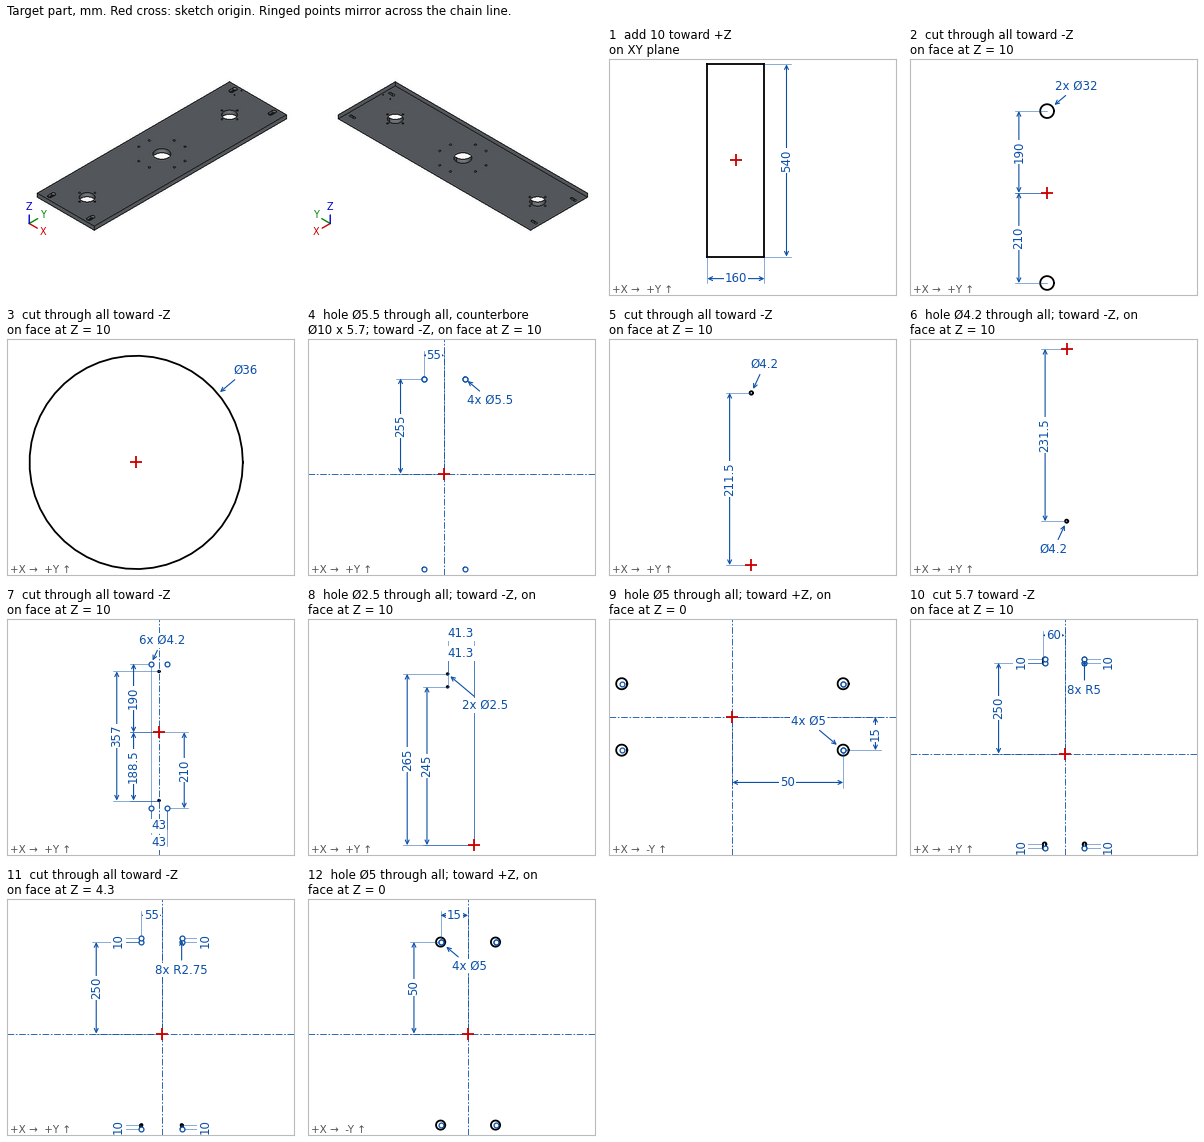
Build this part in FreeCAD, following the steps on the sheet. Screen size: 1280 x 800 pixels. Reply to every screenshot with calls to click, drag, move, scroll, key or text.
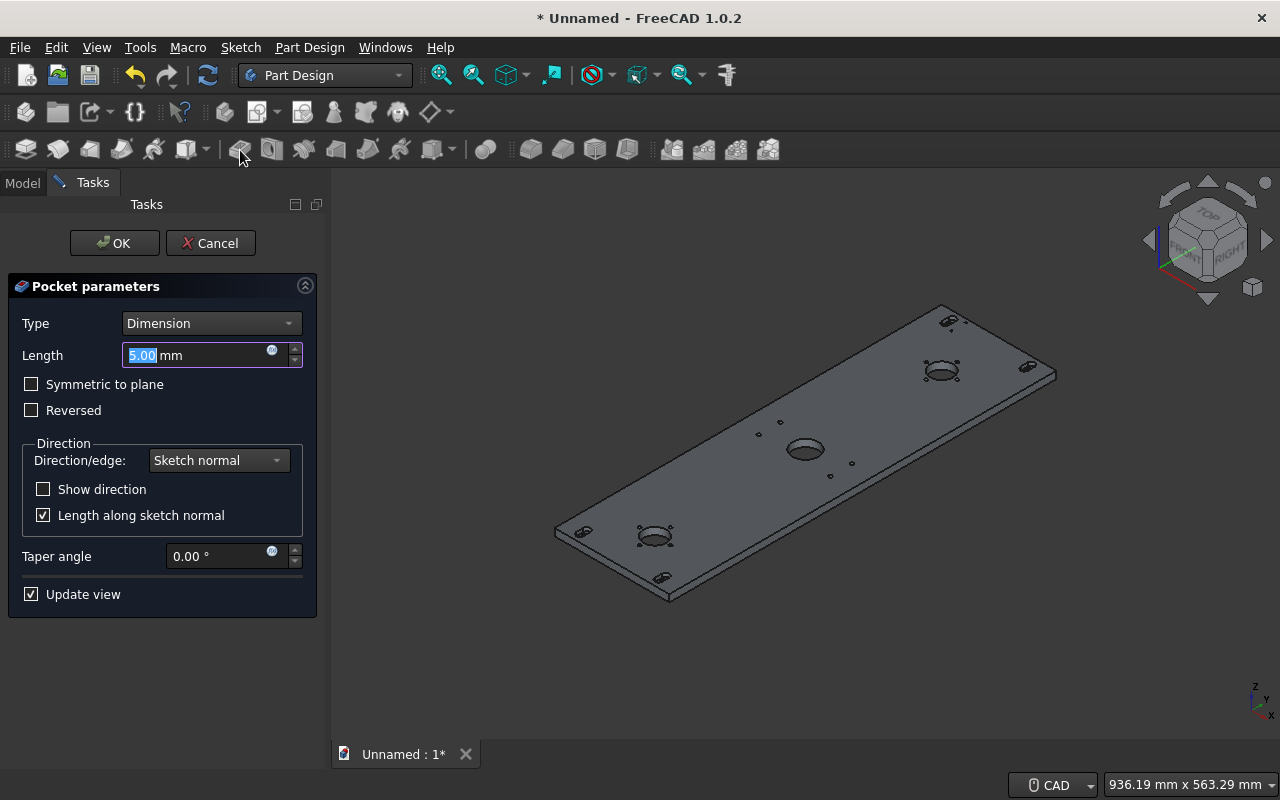
text(5.7)
key(Tab)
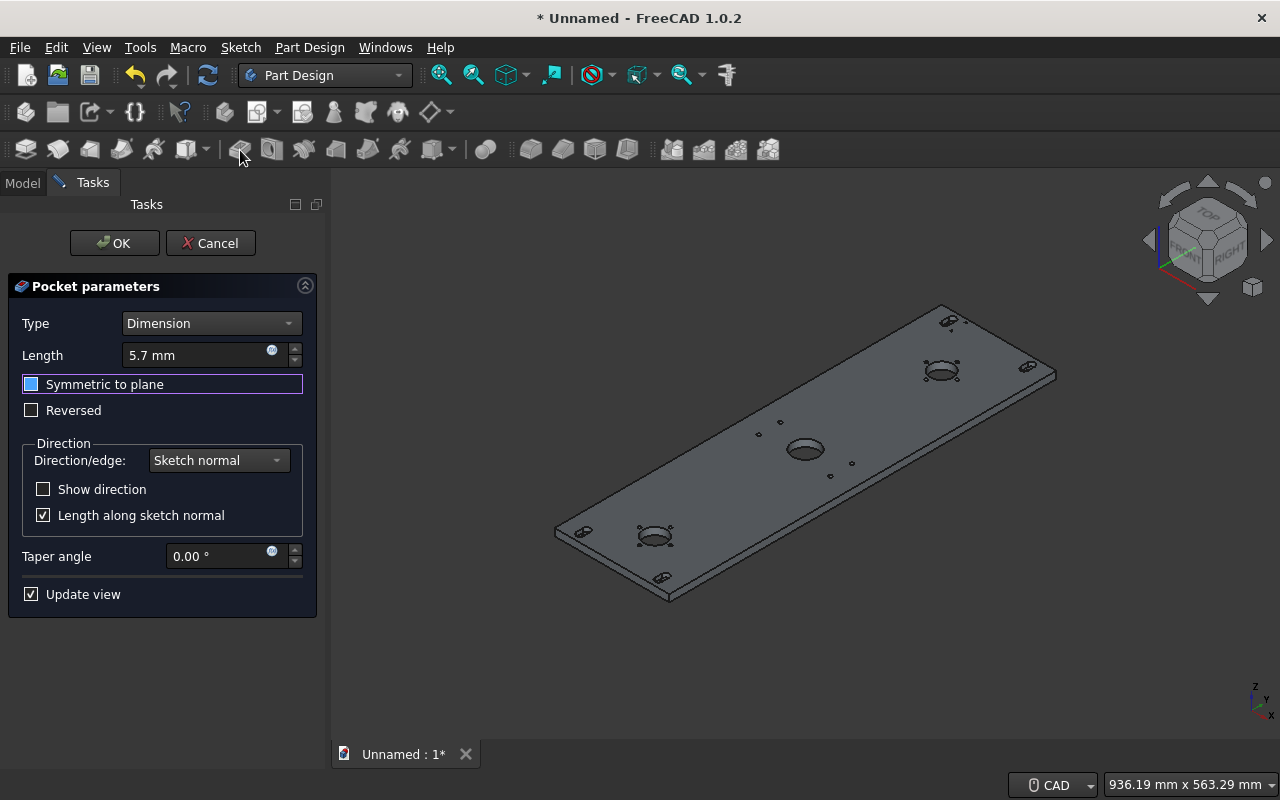
click(115, 243)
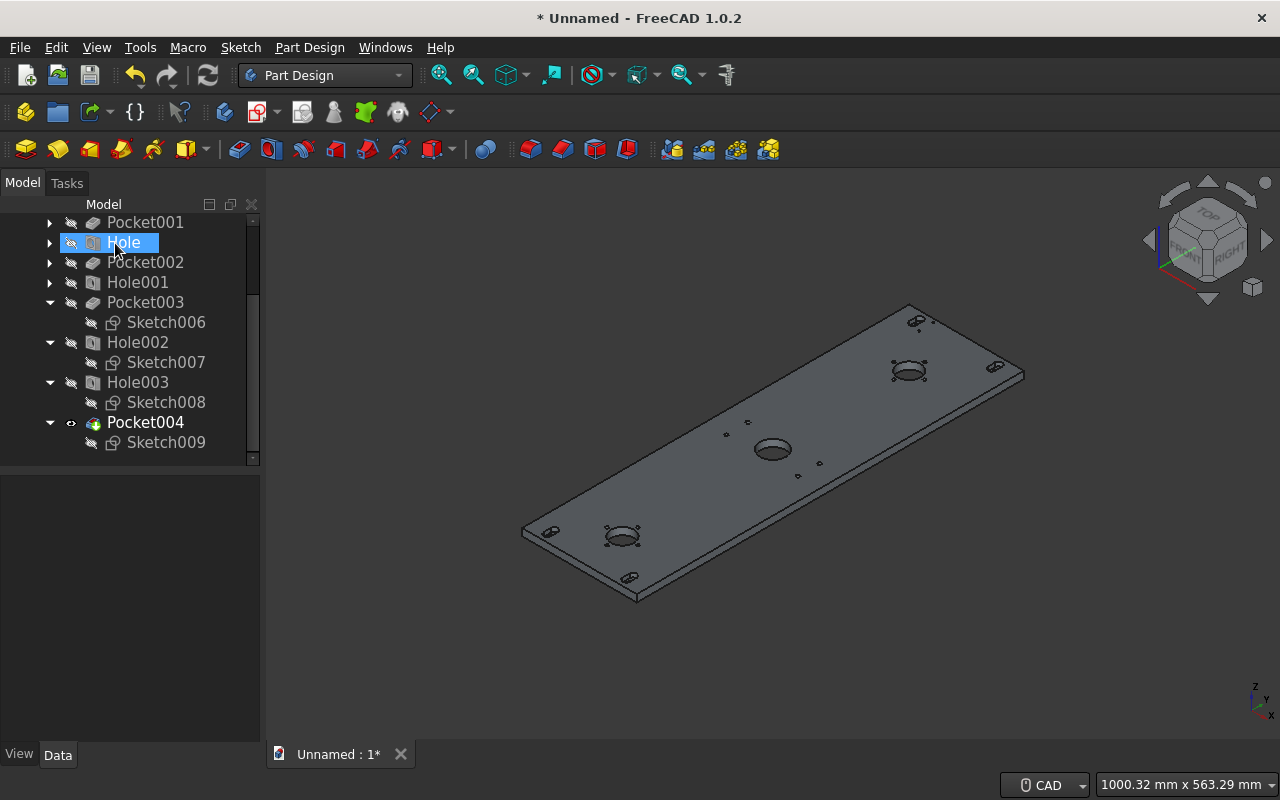
scroll(913, 328, up, 7)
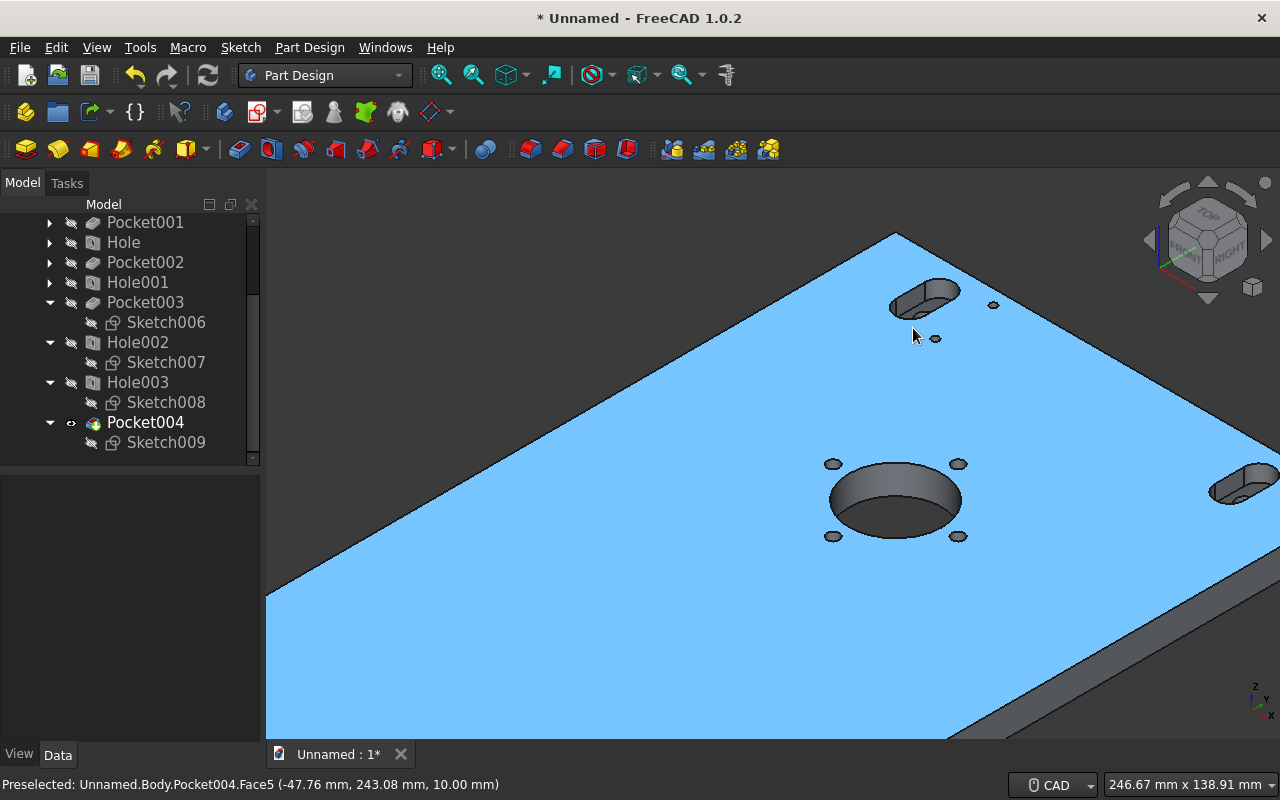
click(442, 76)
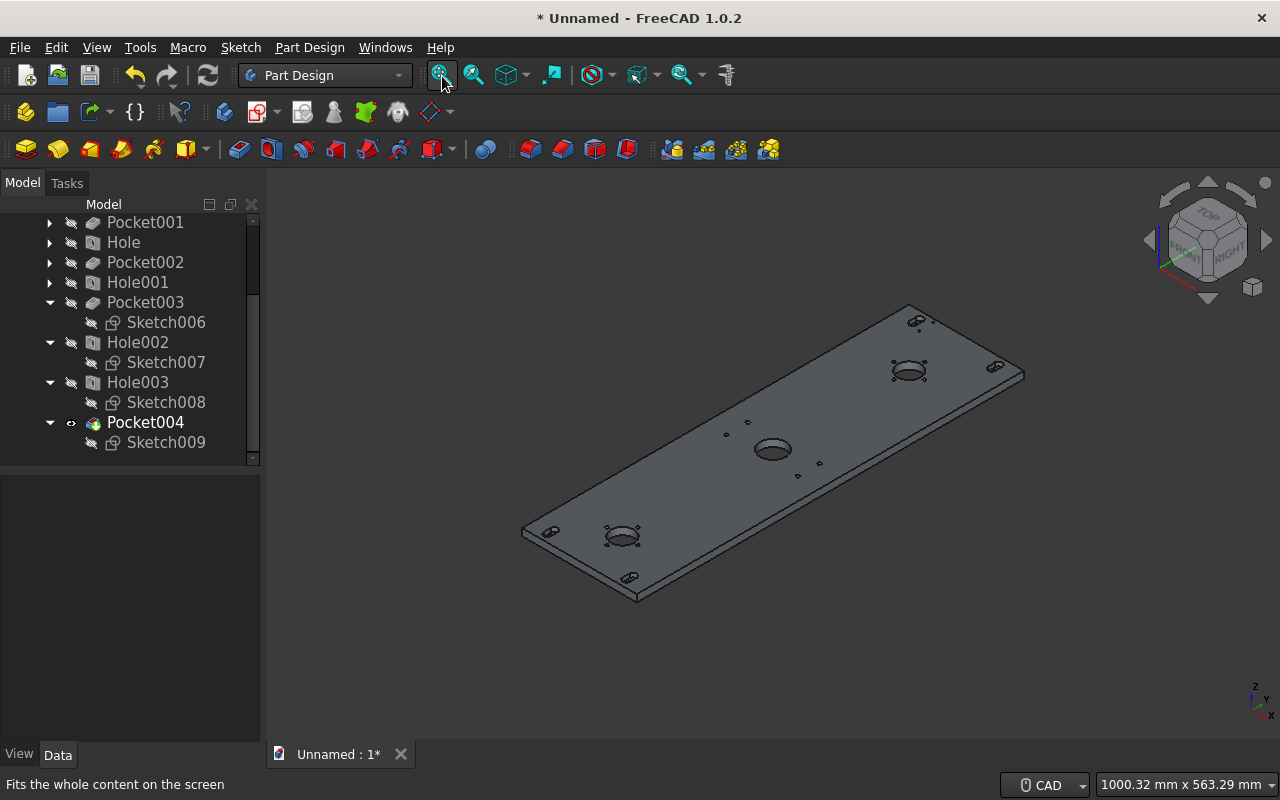
key(2)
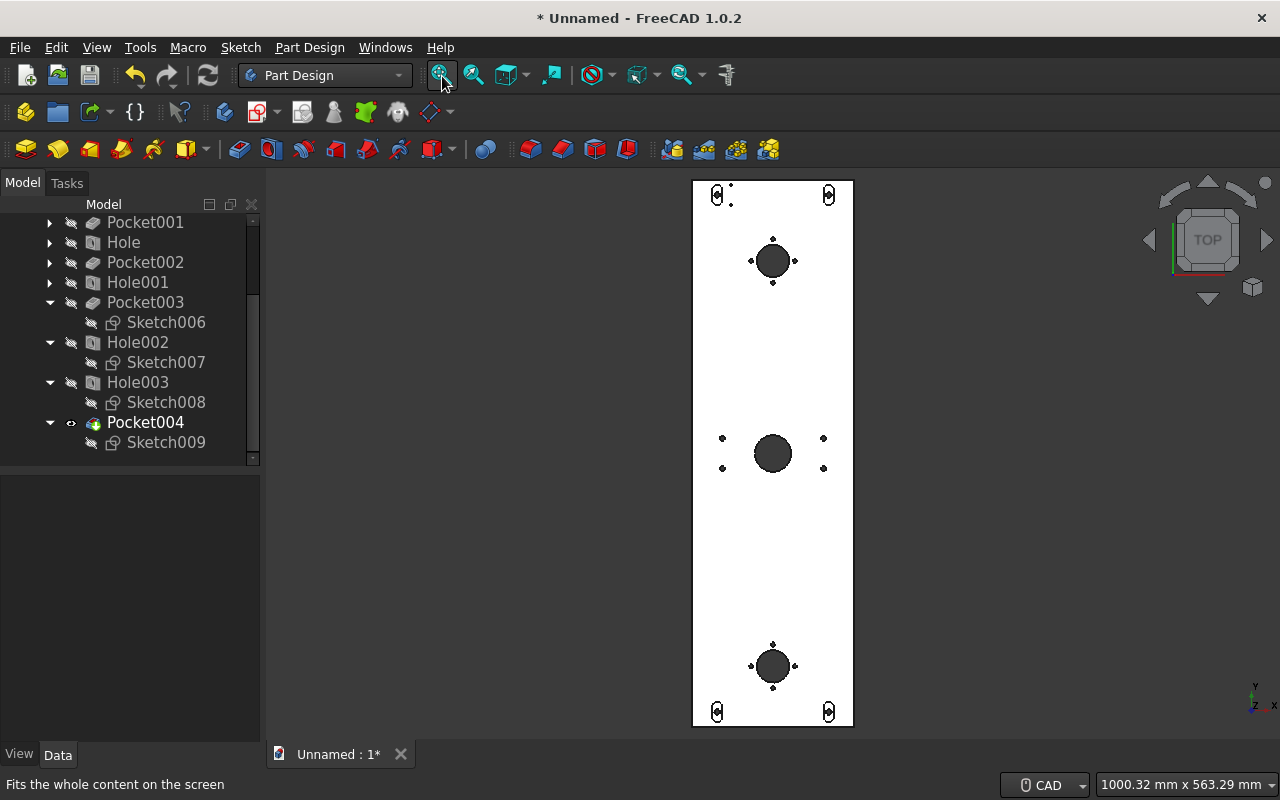
scroll(719, 200, up, 7)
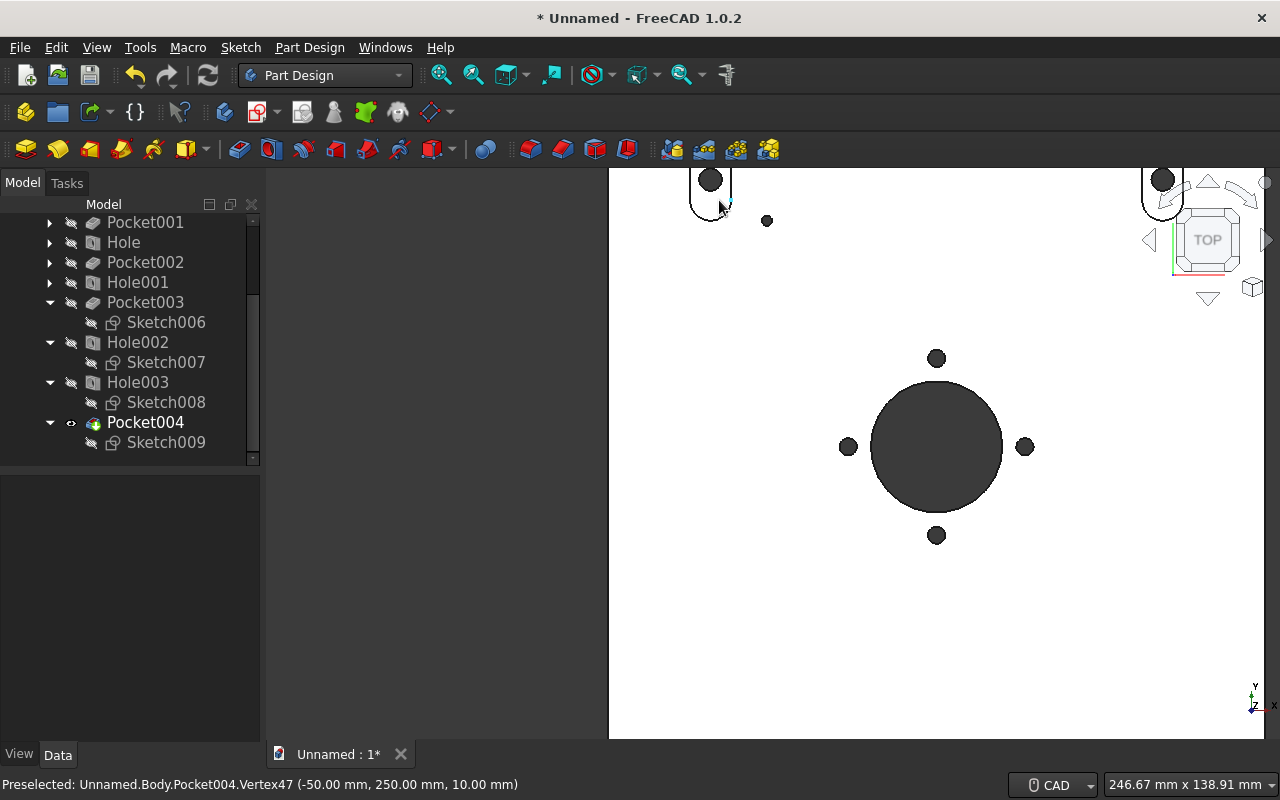
click(716, 202)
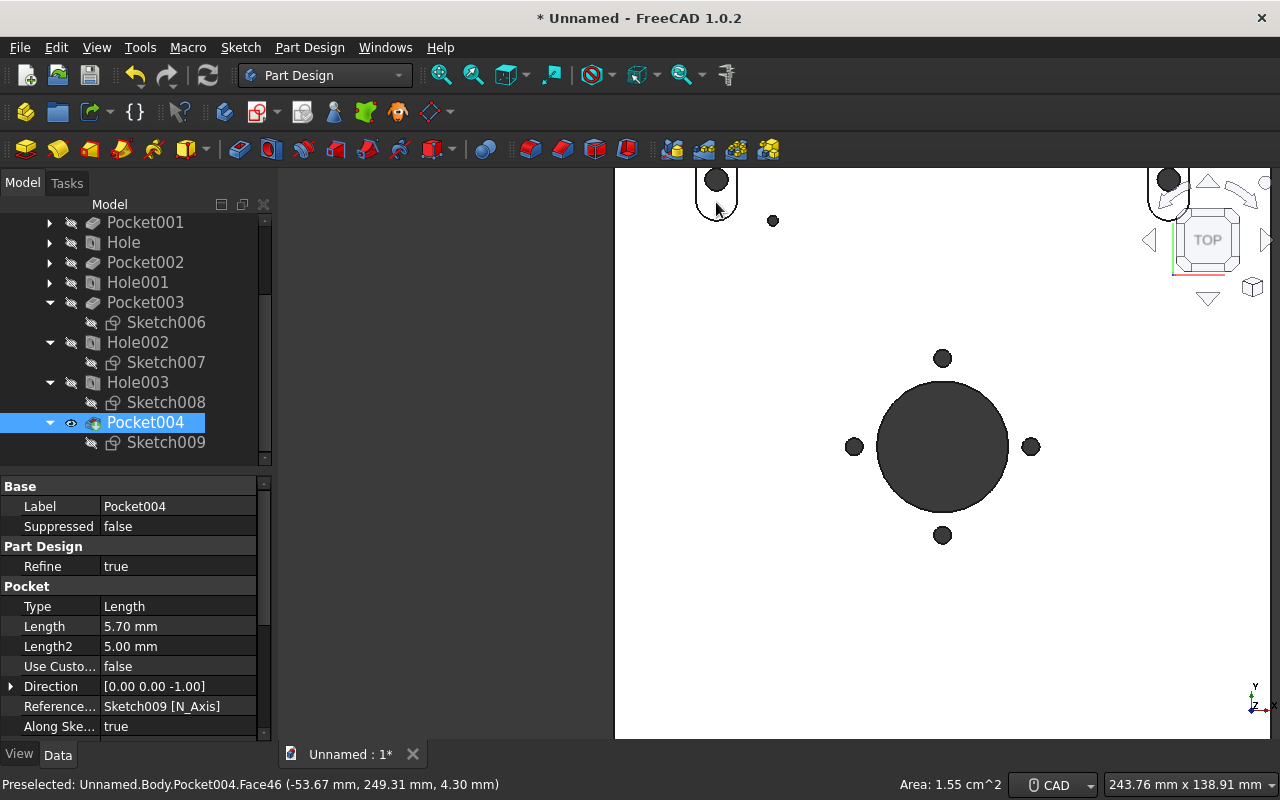
click(258, 112)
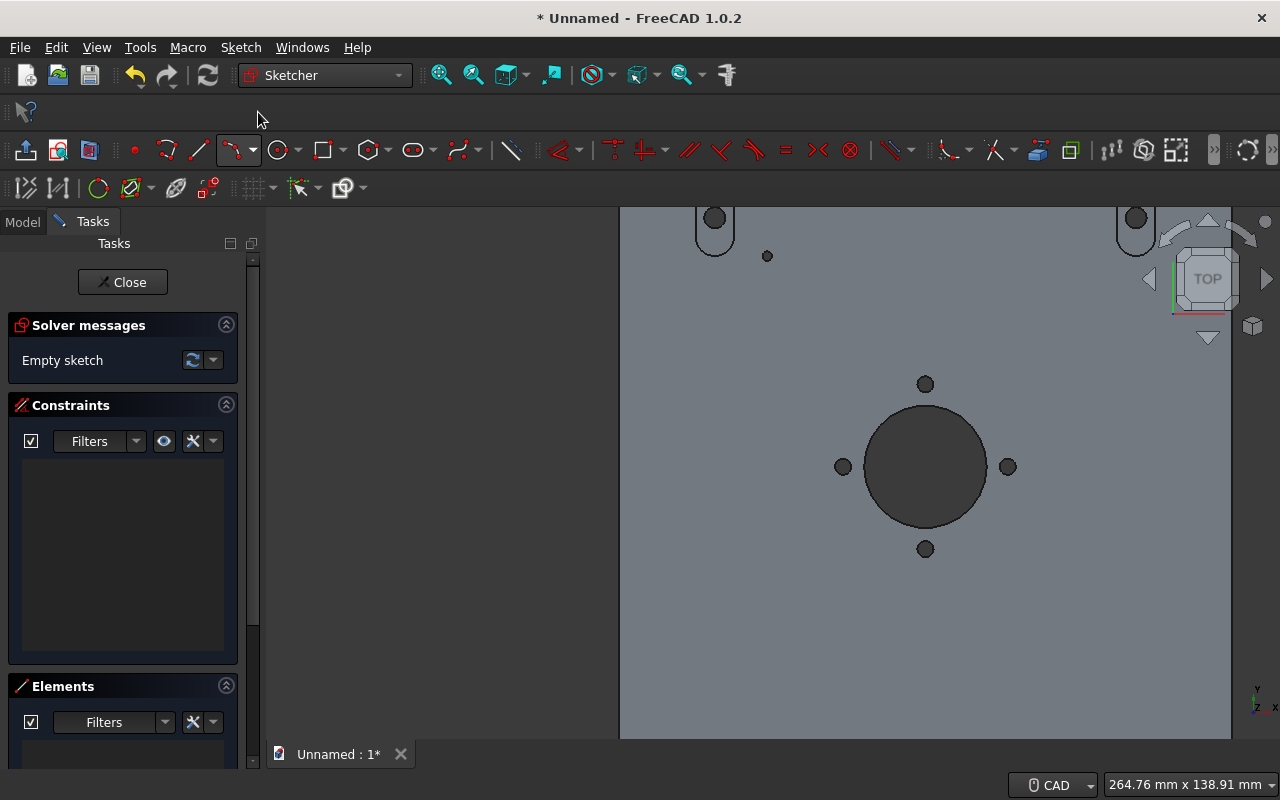
key(q)
key(s)